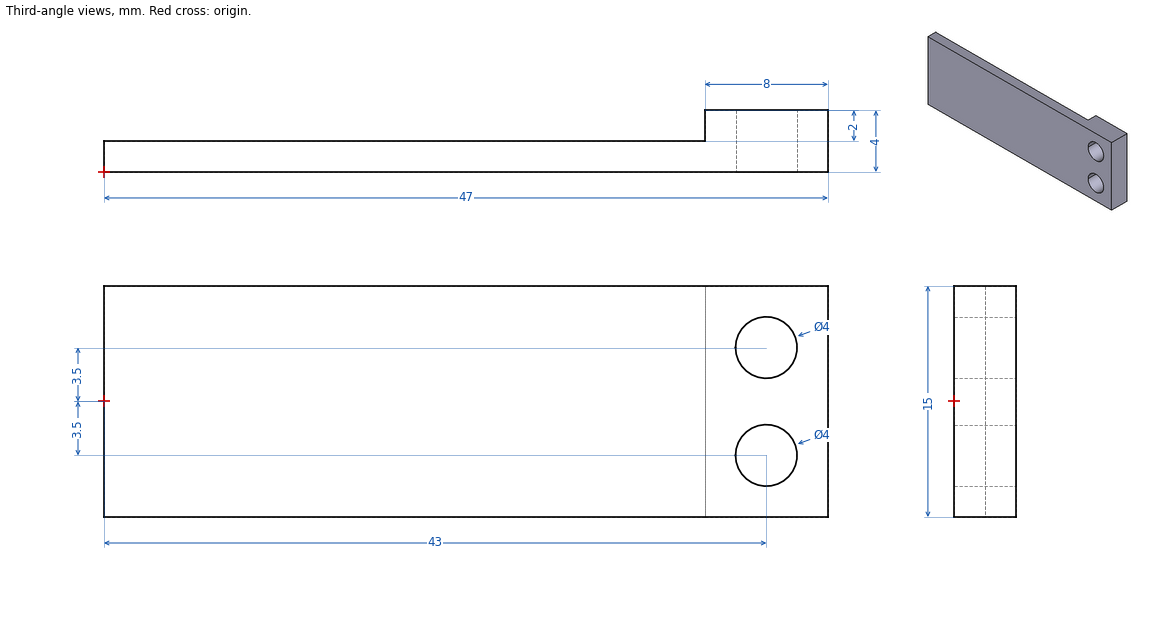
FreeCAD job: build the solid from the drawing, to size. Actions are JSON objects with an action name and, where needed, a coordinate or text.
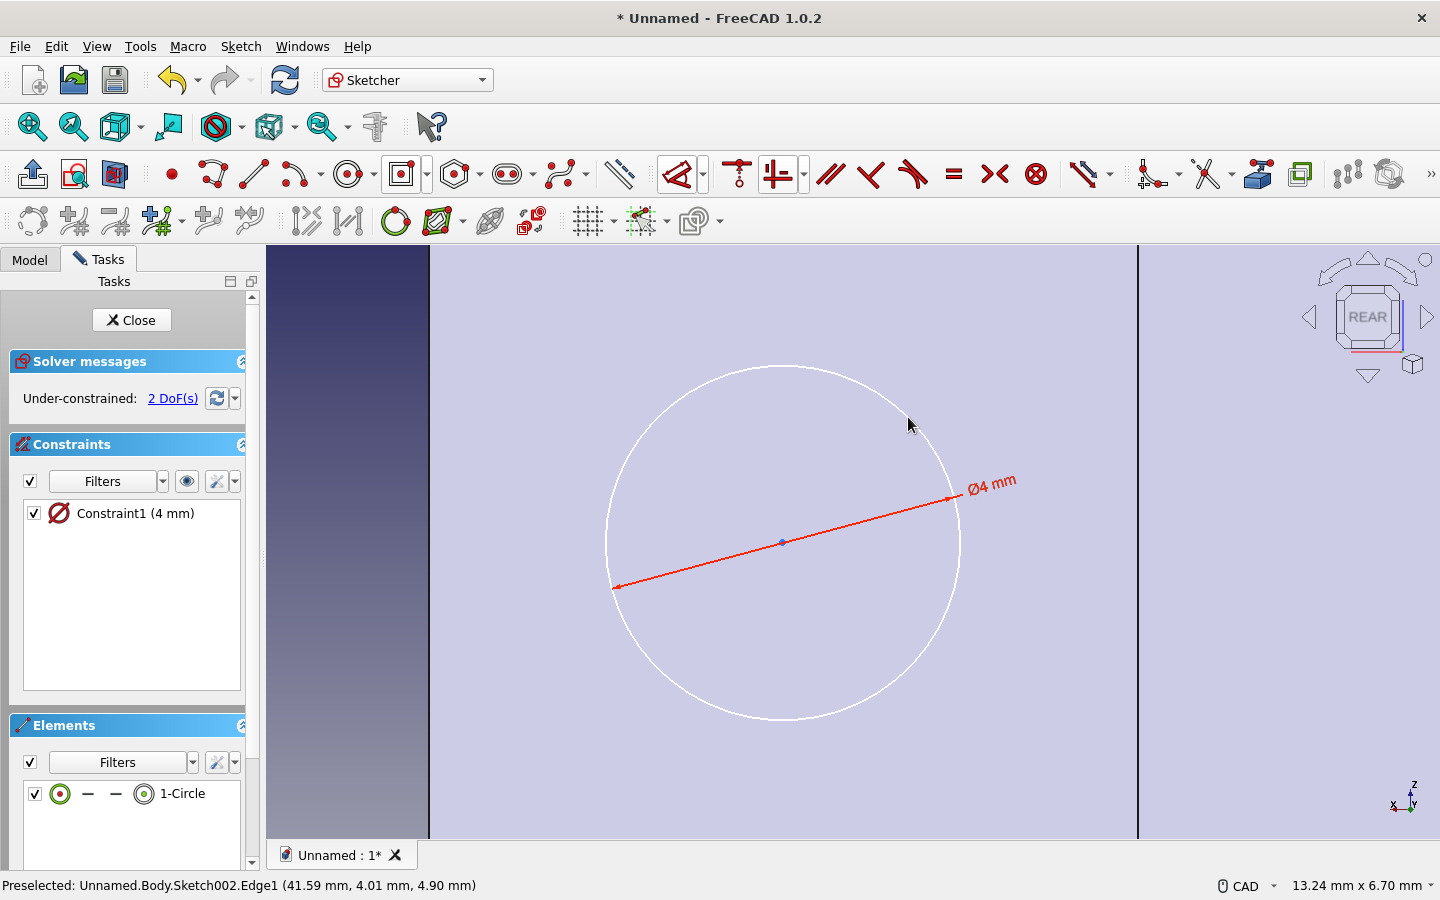
{"action": "left_click", "coordinate": [783, 543]}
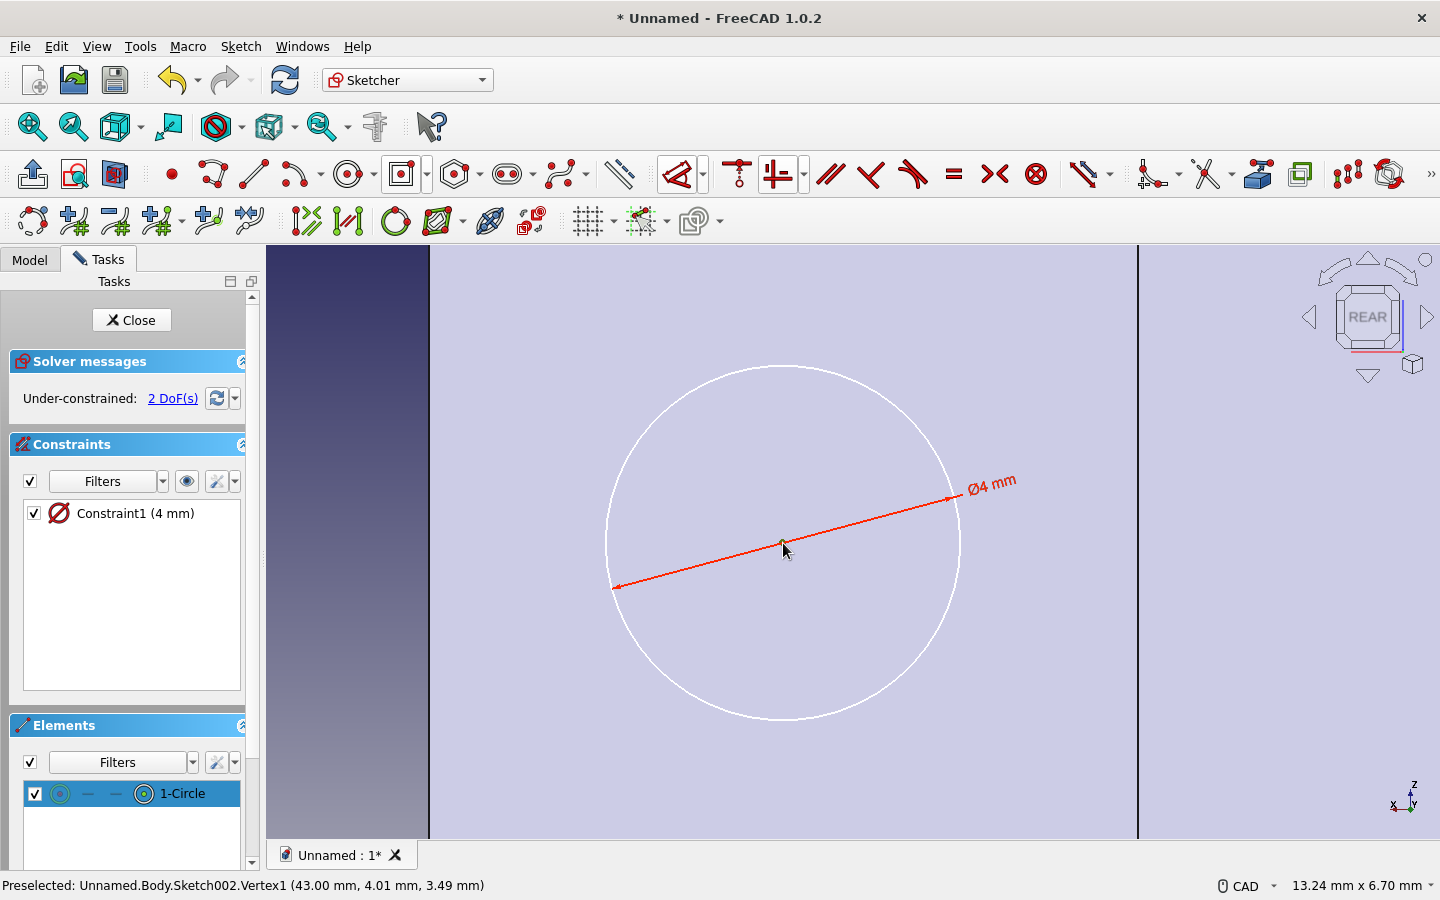
{"action": "key", "text": "l"}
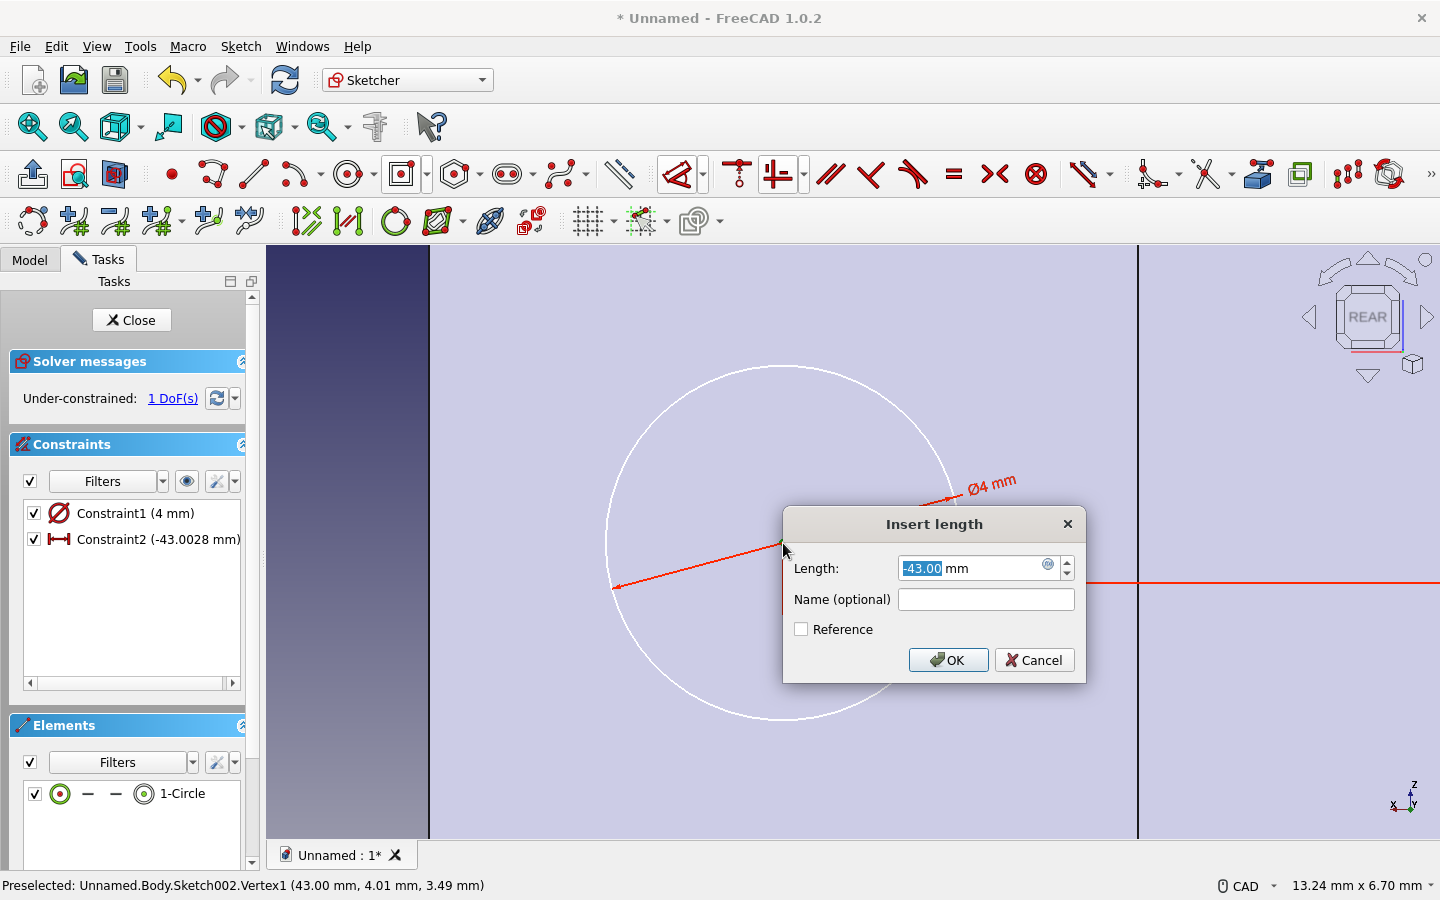
{"action": "type", "text": "-43"}
{"action": "key", "text": "Return"}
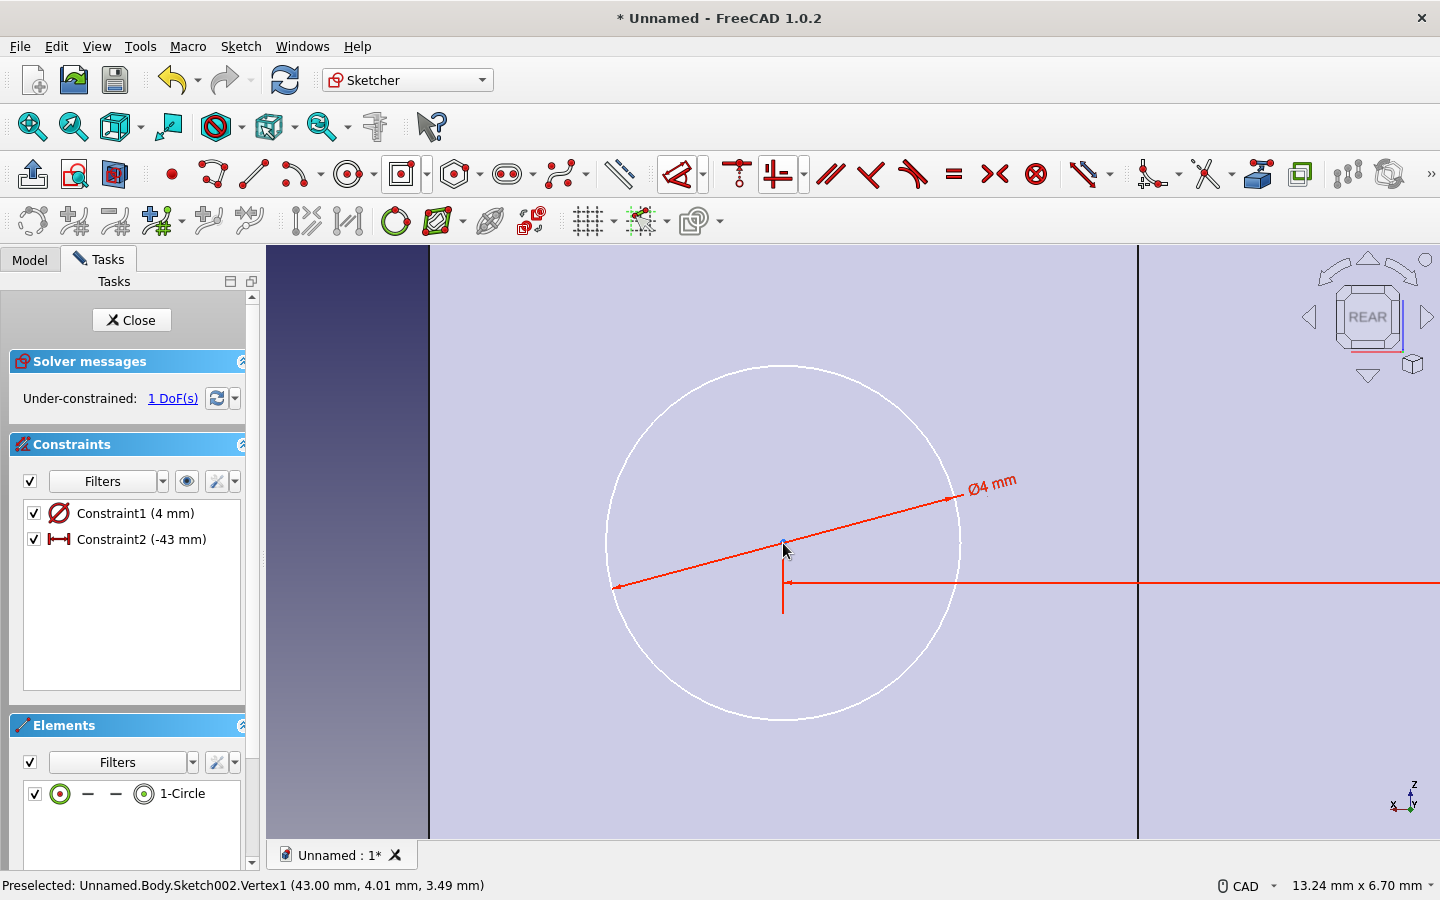
{"action": "left_click", "coordinate": [783, 543]}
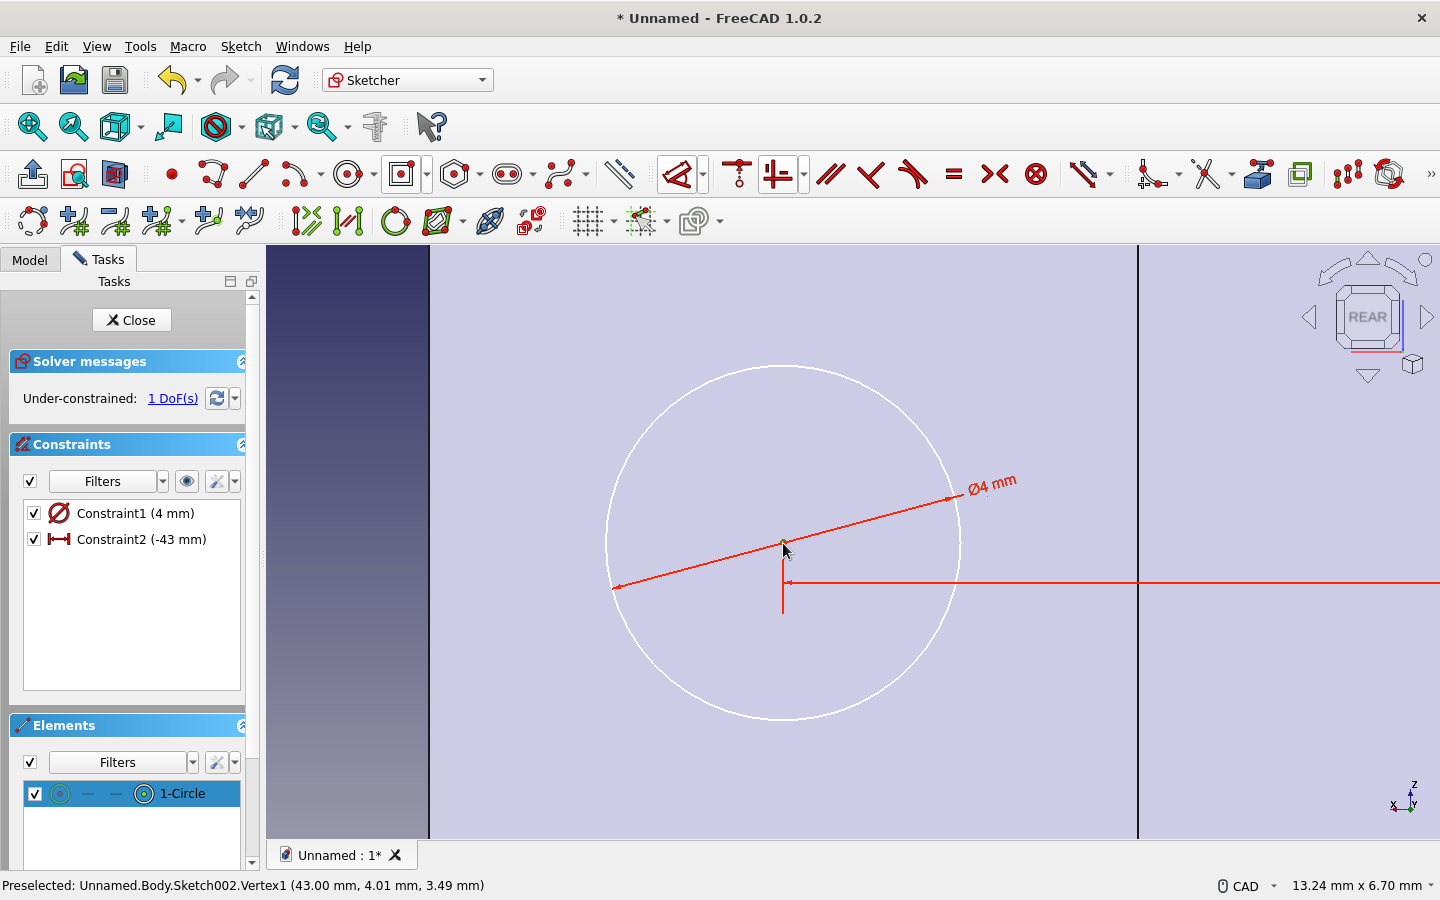
{"action": "key", "text": "i"}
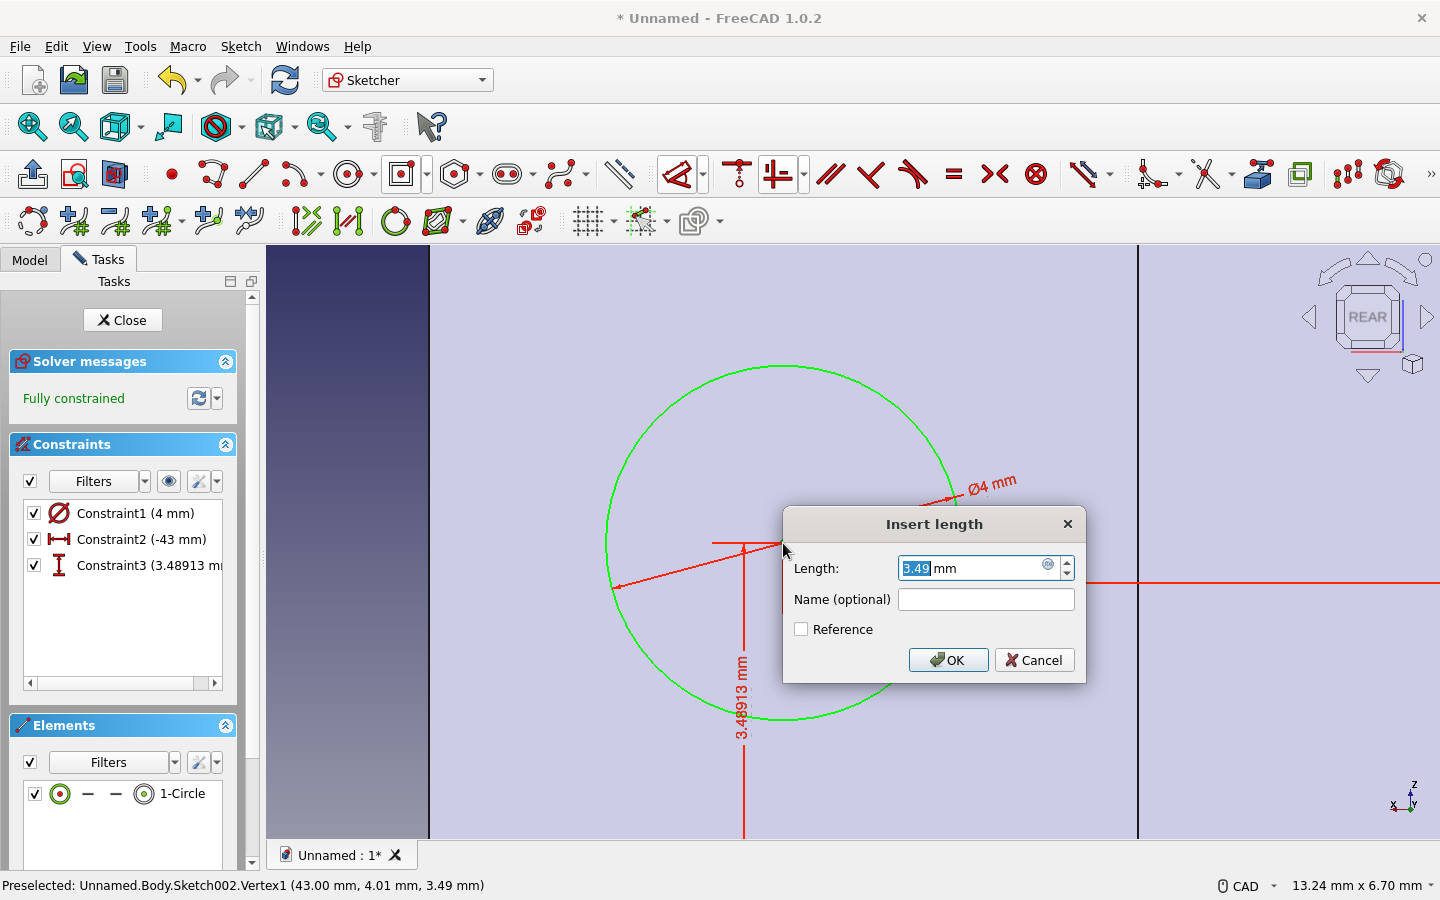
{"action": "type", "text": "3.5"}
{"action": "key", "text": "Return"}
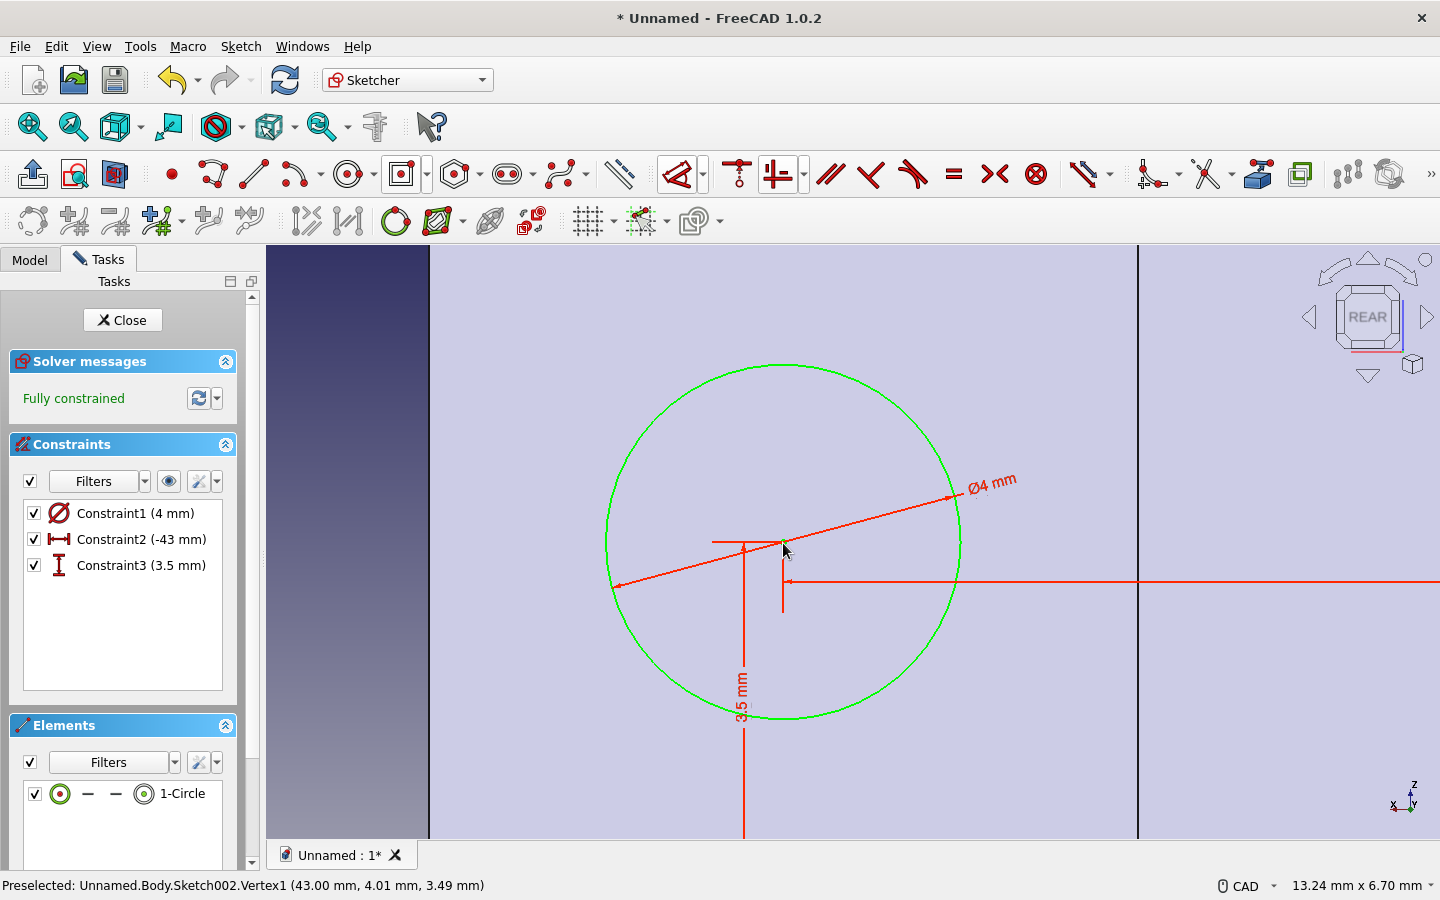
{"action": "left_click", "coordinate": [123, 320]}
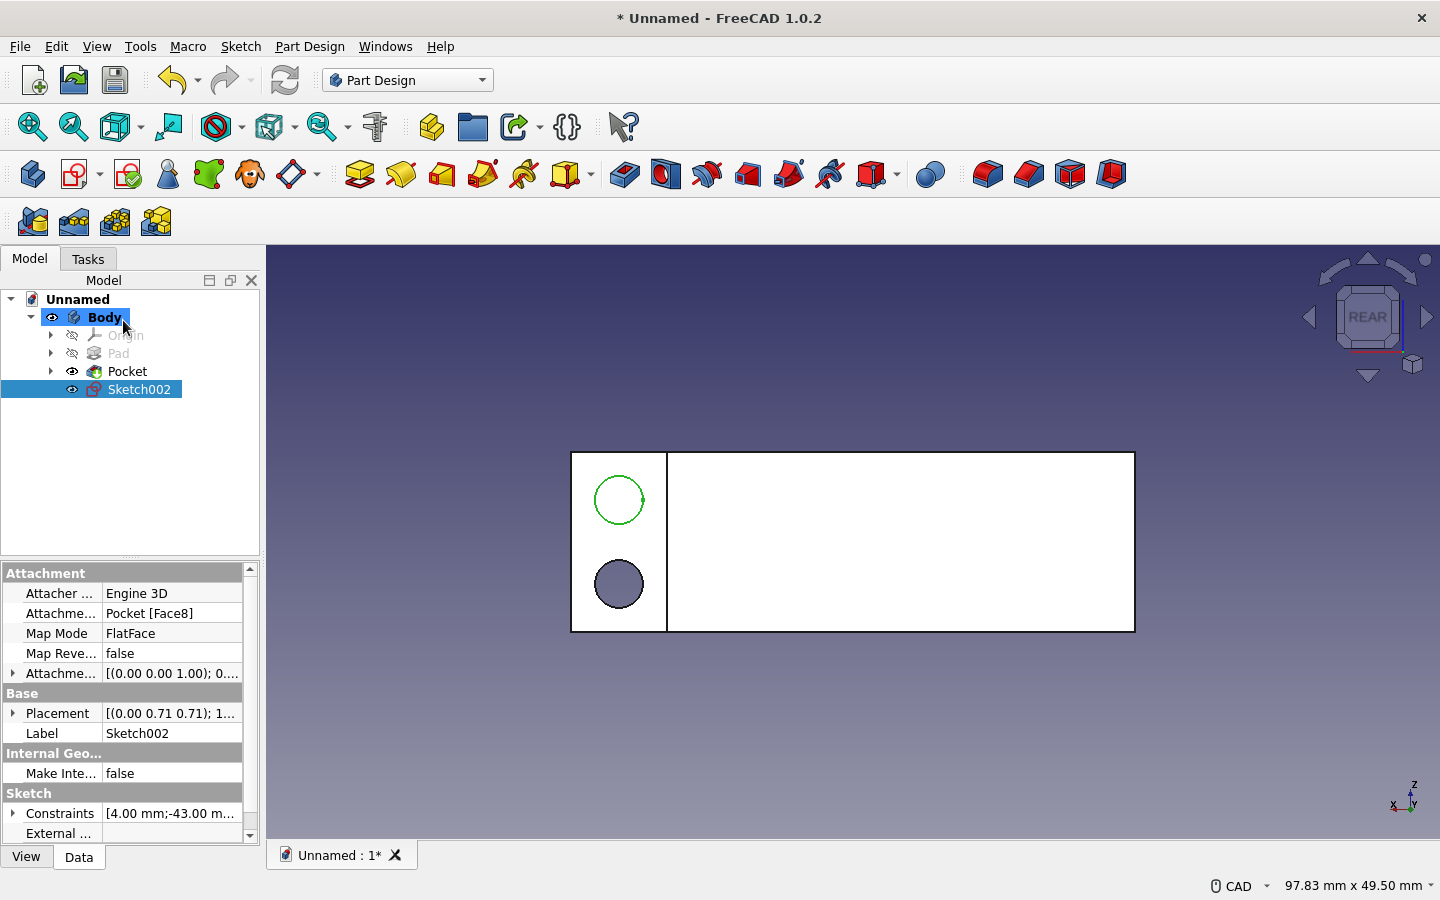
{"action": "left_click", "coordinate": [625, 174]}